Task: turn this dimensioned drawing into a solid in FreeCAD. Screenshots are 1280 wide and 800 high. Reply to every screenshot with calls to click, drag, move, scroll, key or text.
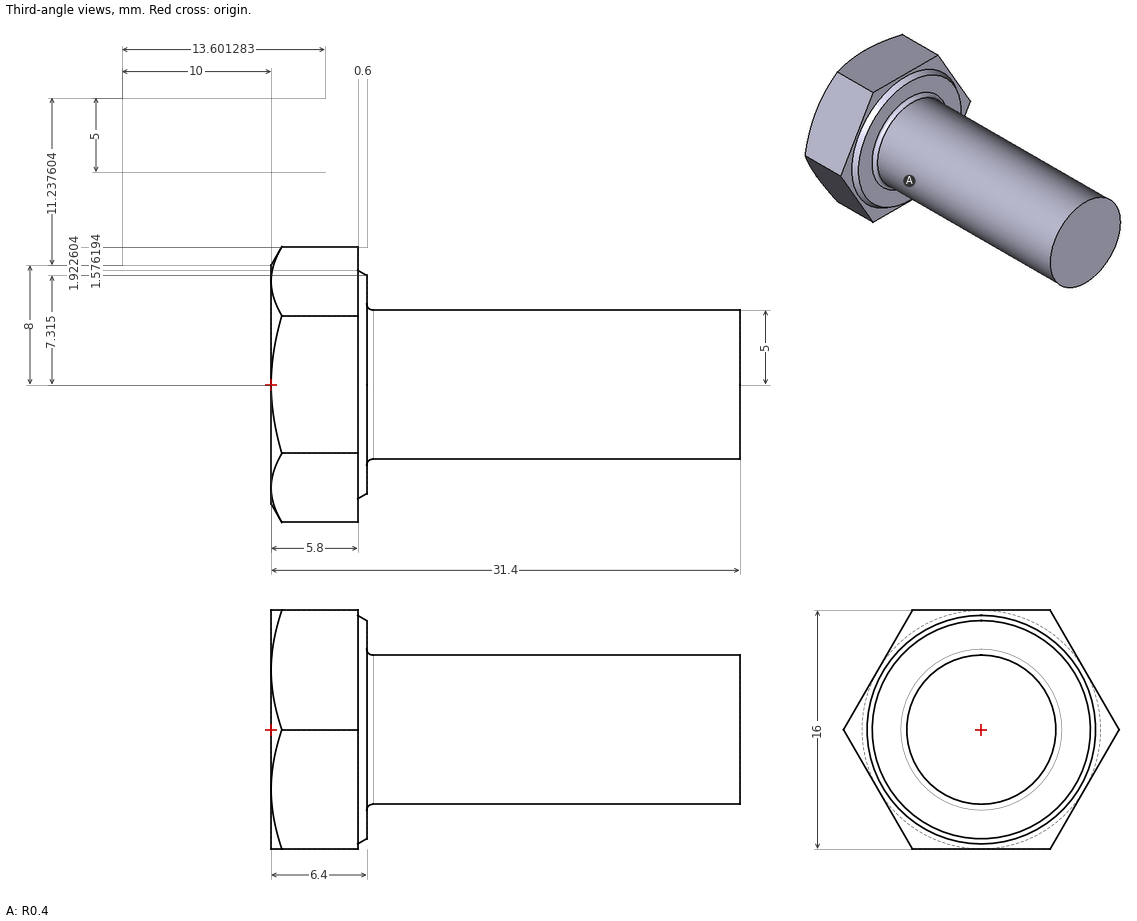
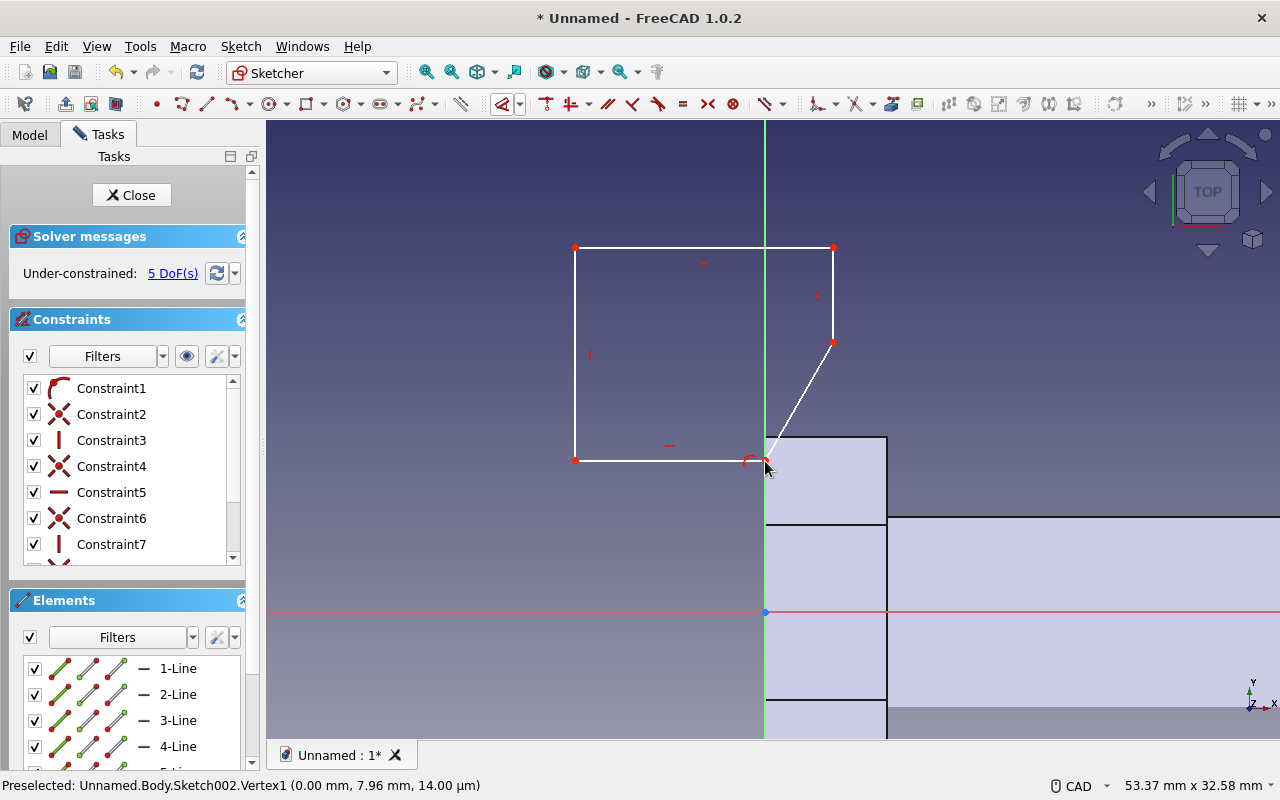
click(833, 315)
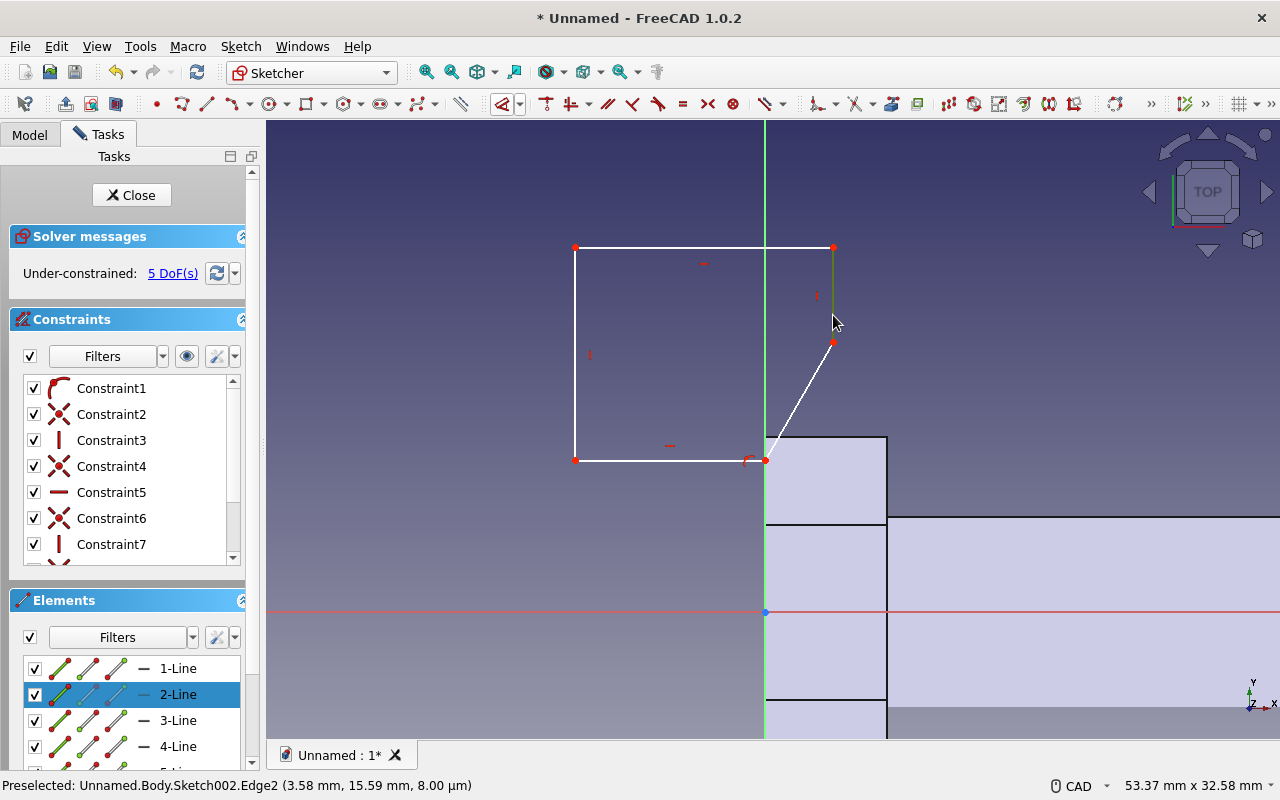
click(520, 104)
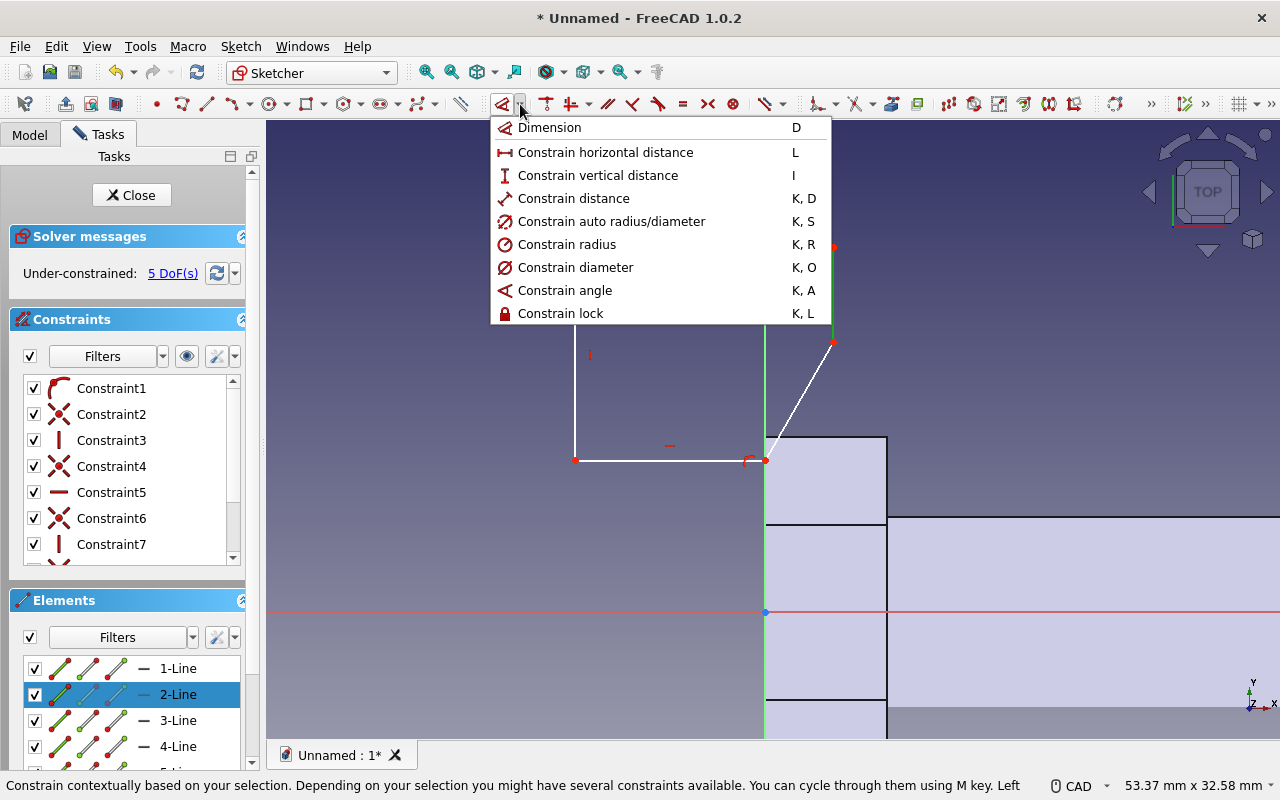
click(661, 176)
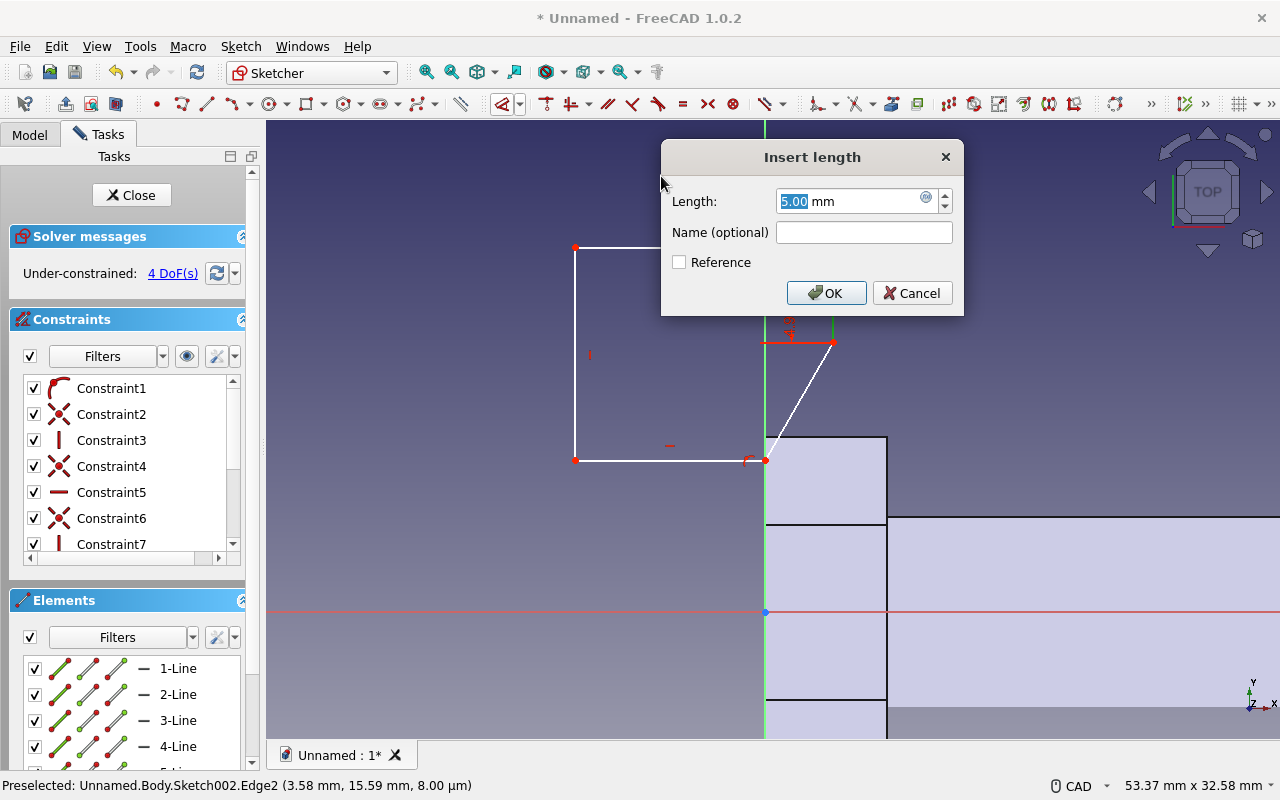
text(5)
key(Return)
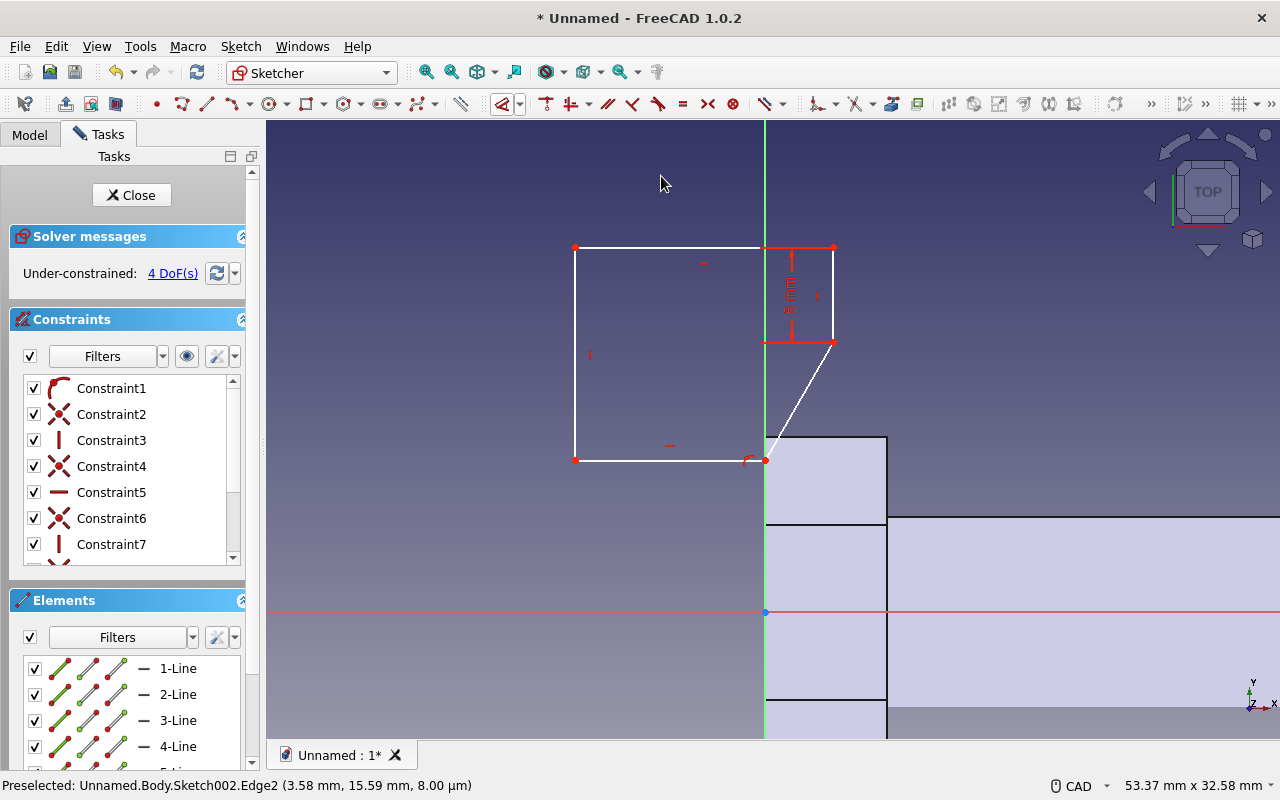
click(632, 461)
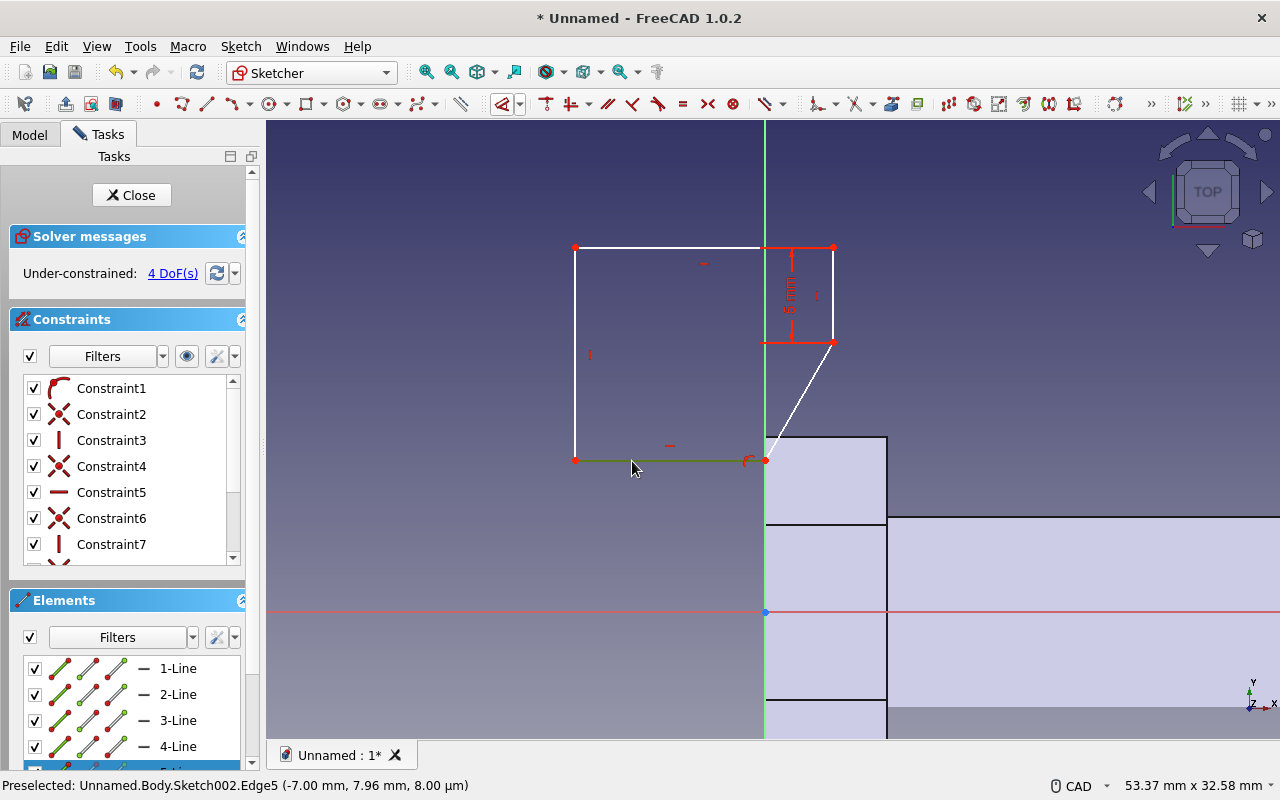
key(l)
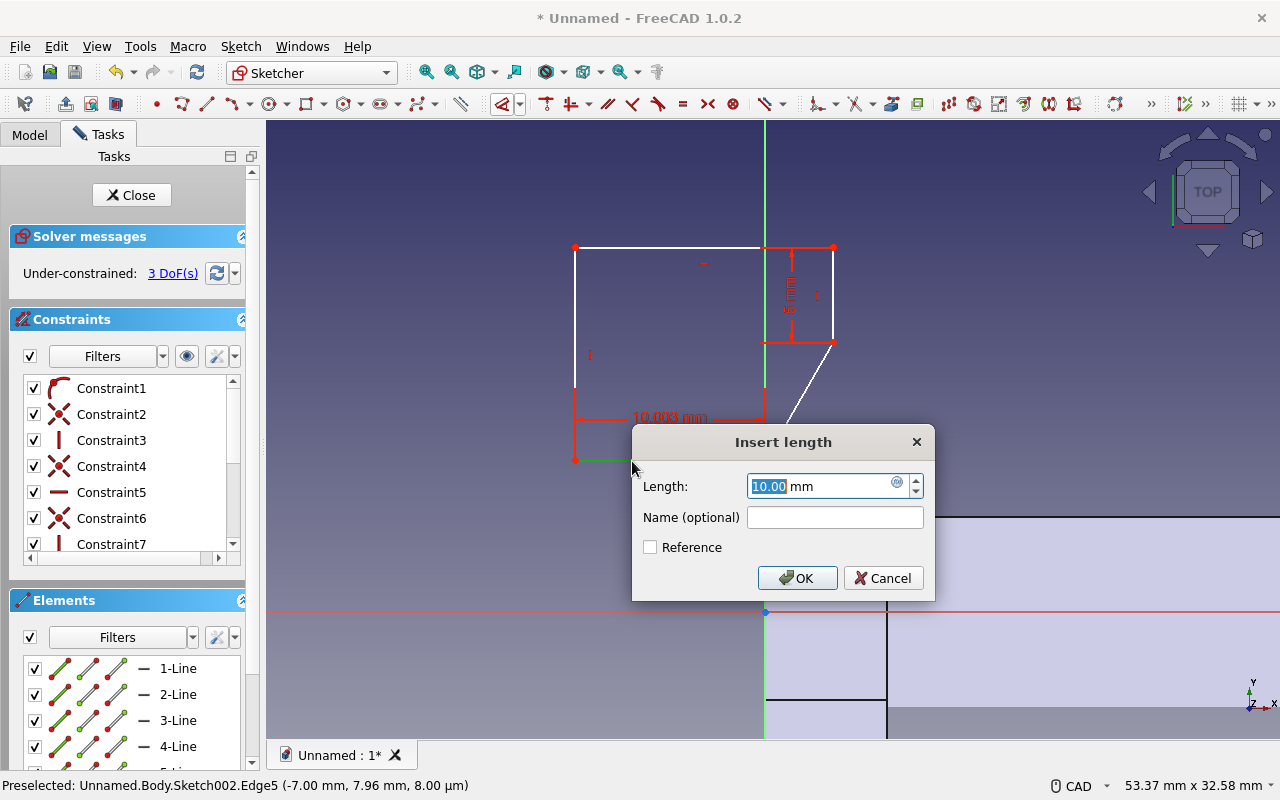
text(10)
key(Return)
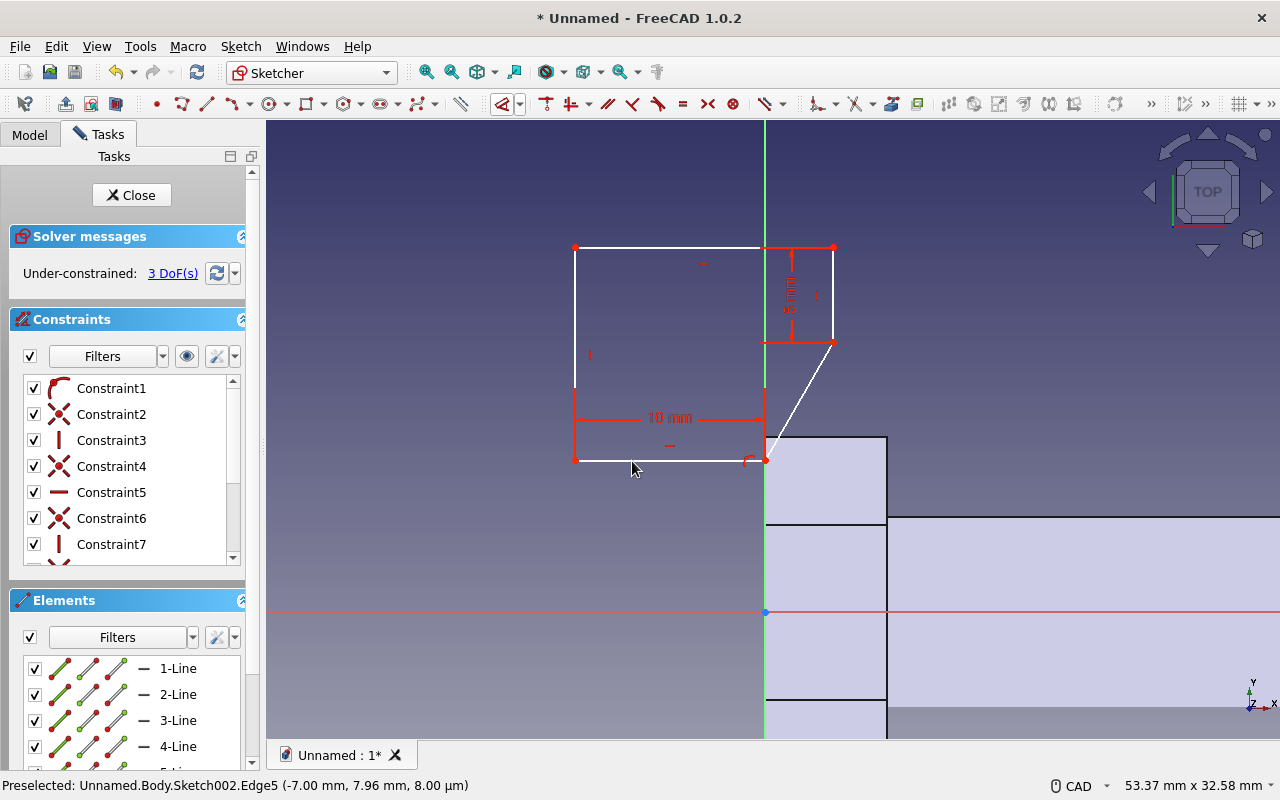
click(765, 461)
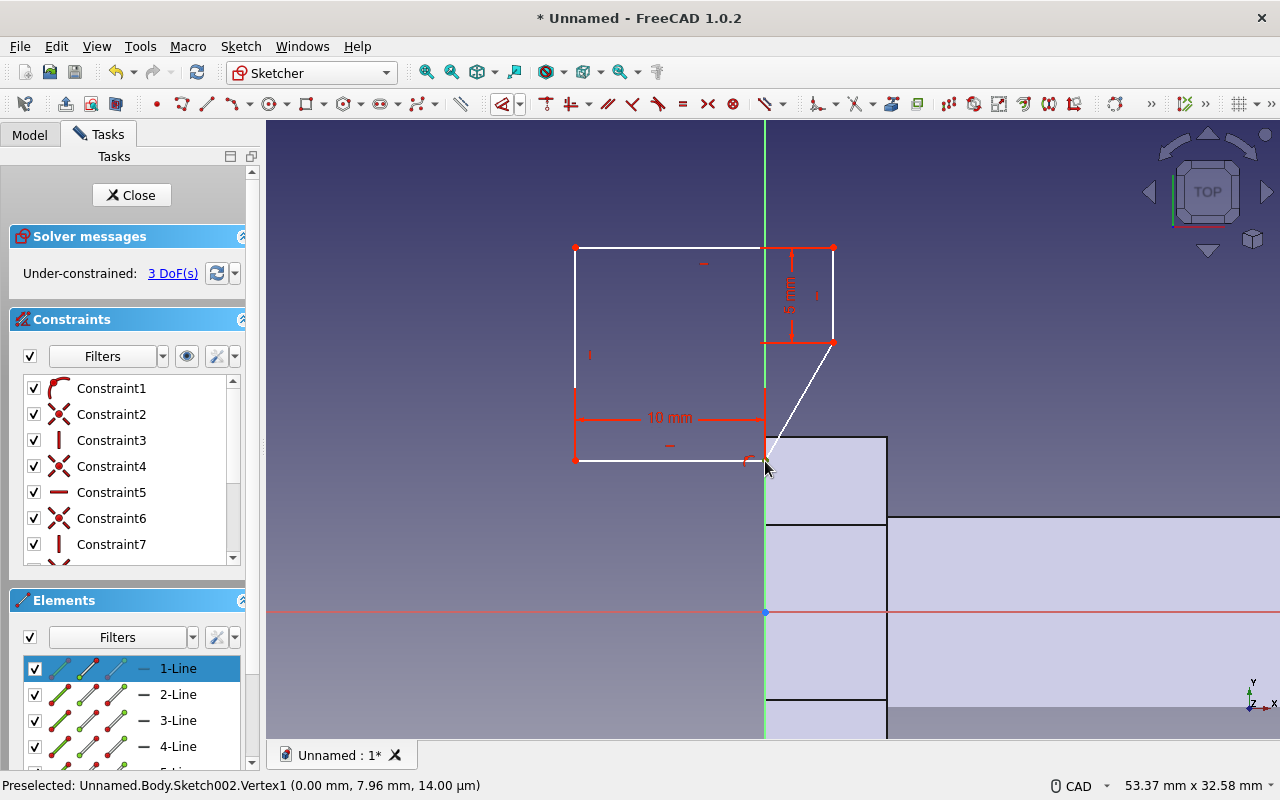
click(520, 104)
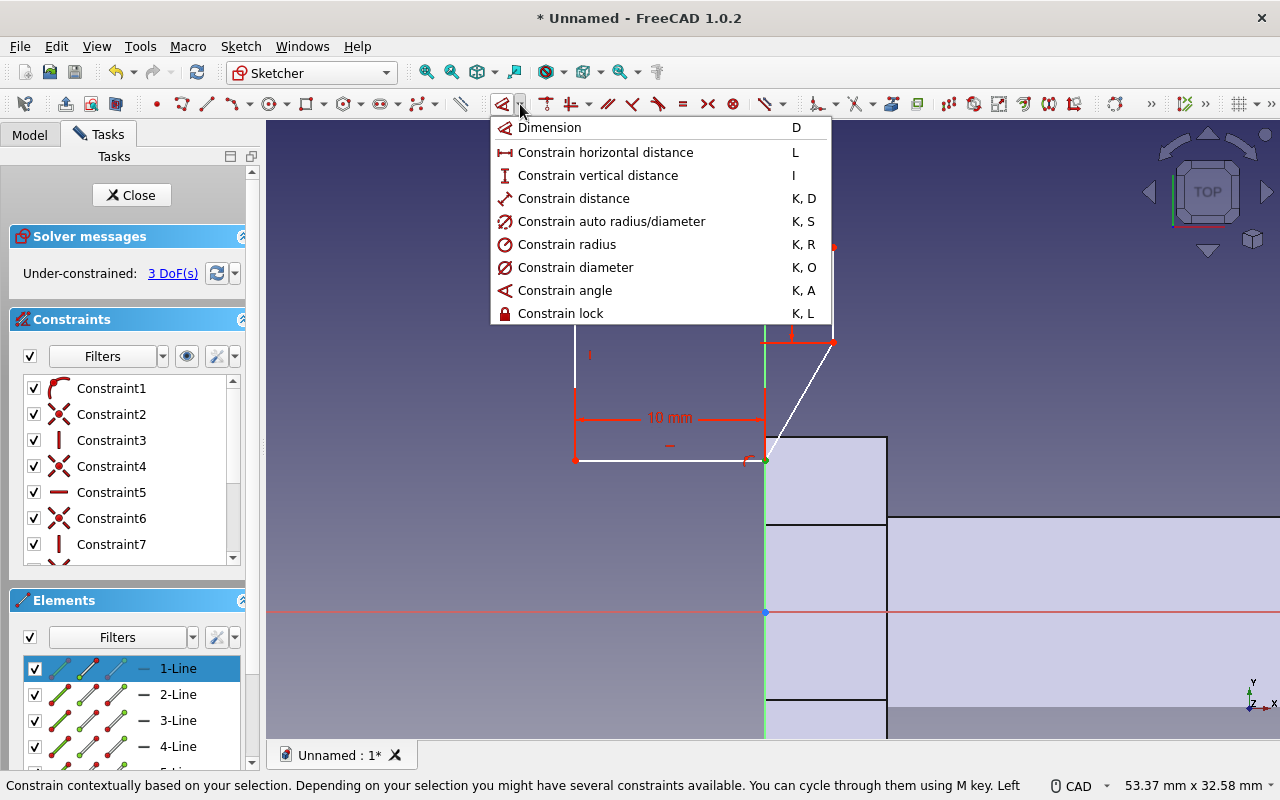
click(661, 176)